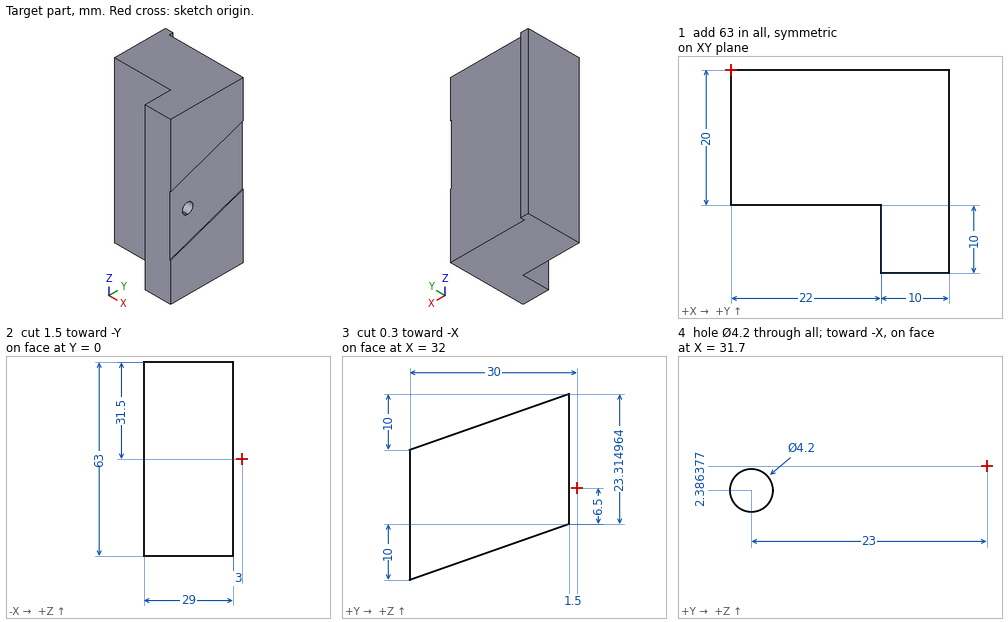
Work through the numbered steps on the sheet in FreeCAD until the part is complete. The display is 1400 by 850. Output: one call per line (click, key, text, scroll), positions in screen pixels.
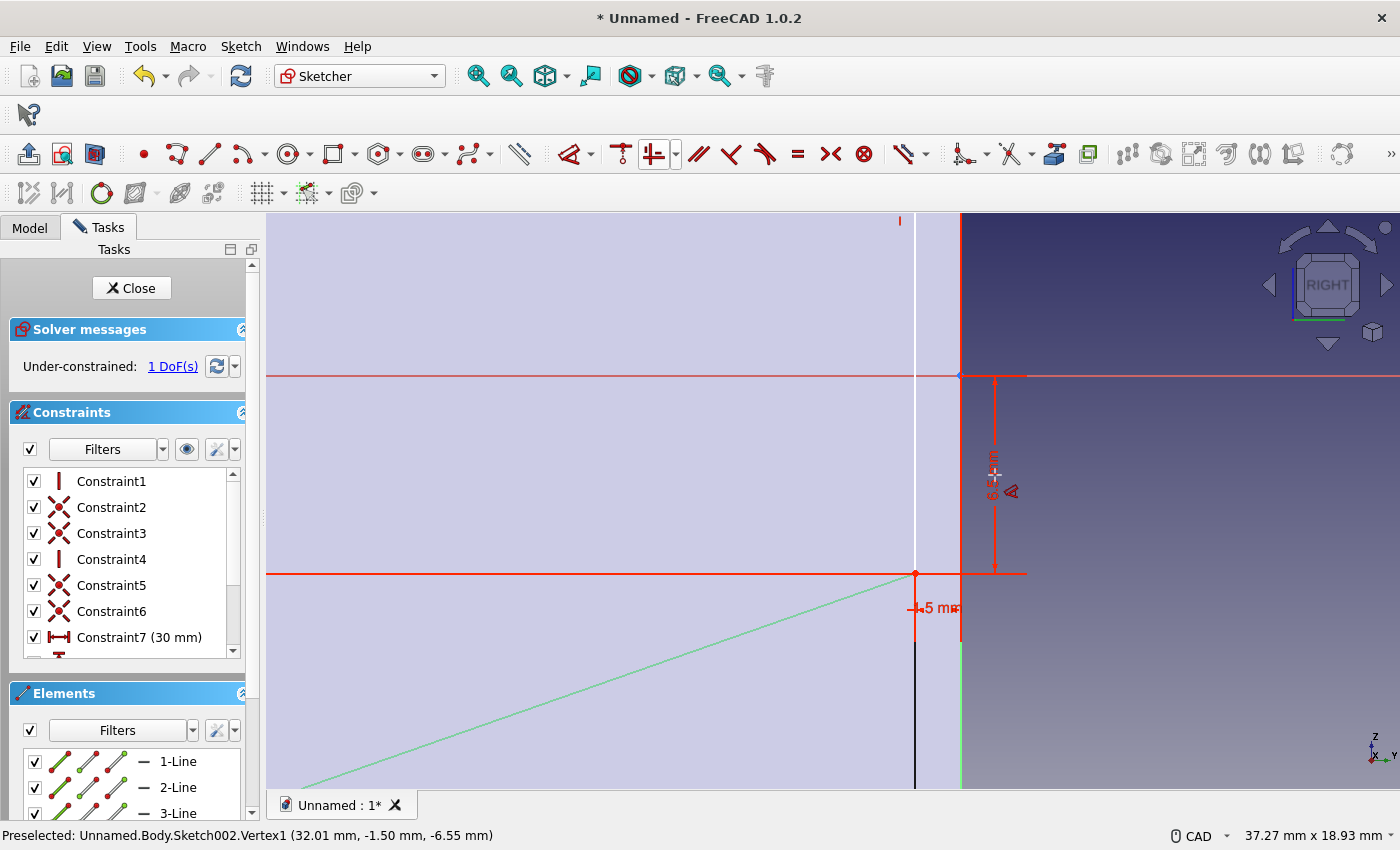
click(915, 362)
click(881, 407)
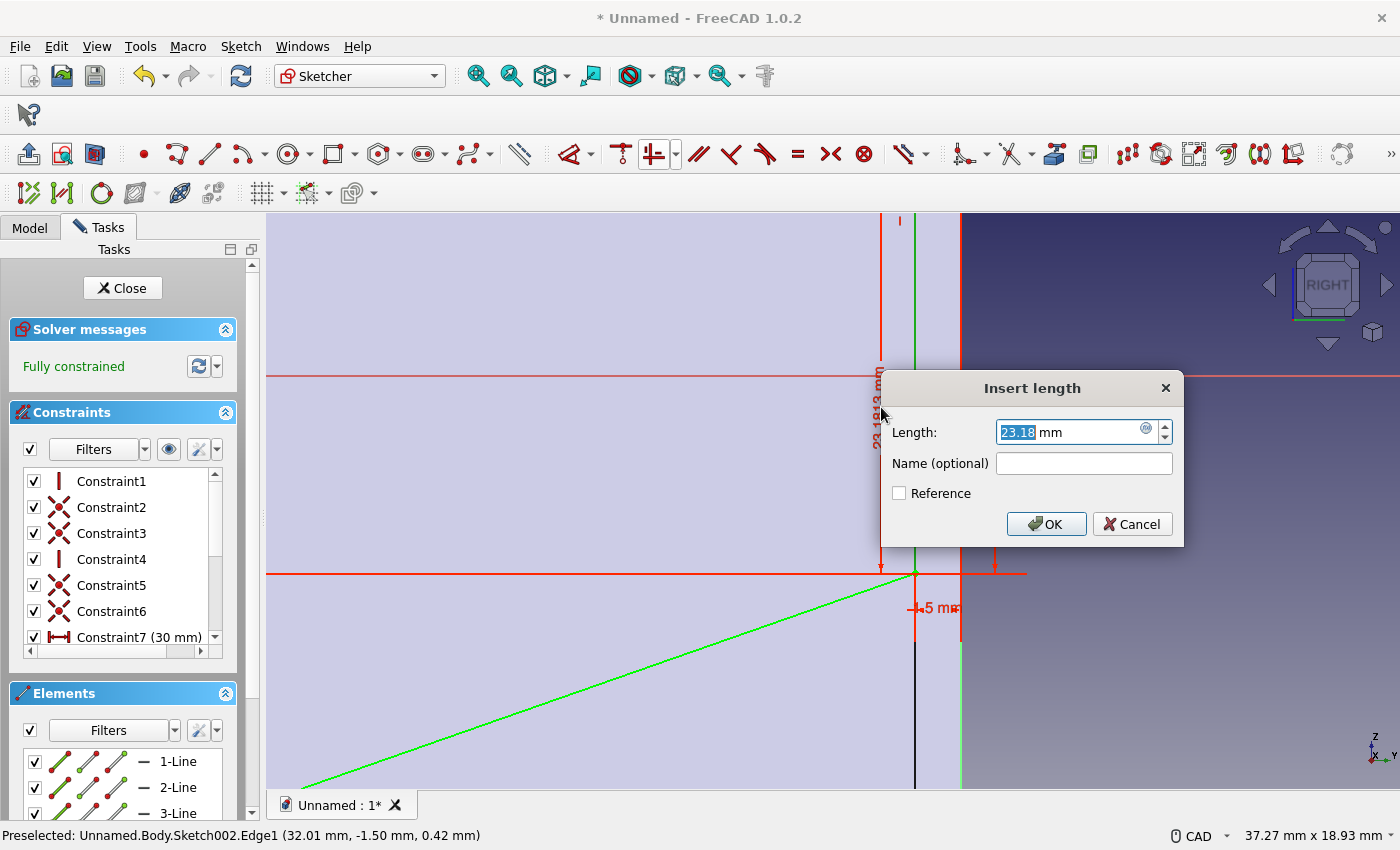
text(23.314964)
key(Return)
key(Escape)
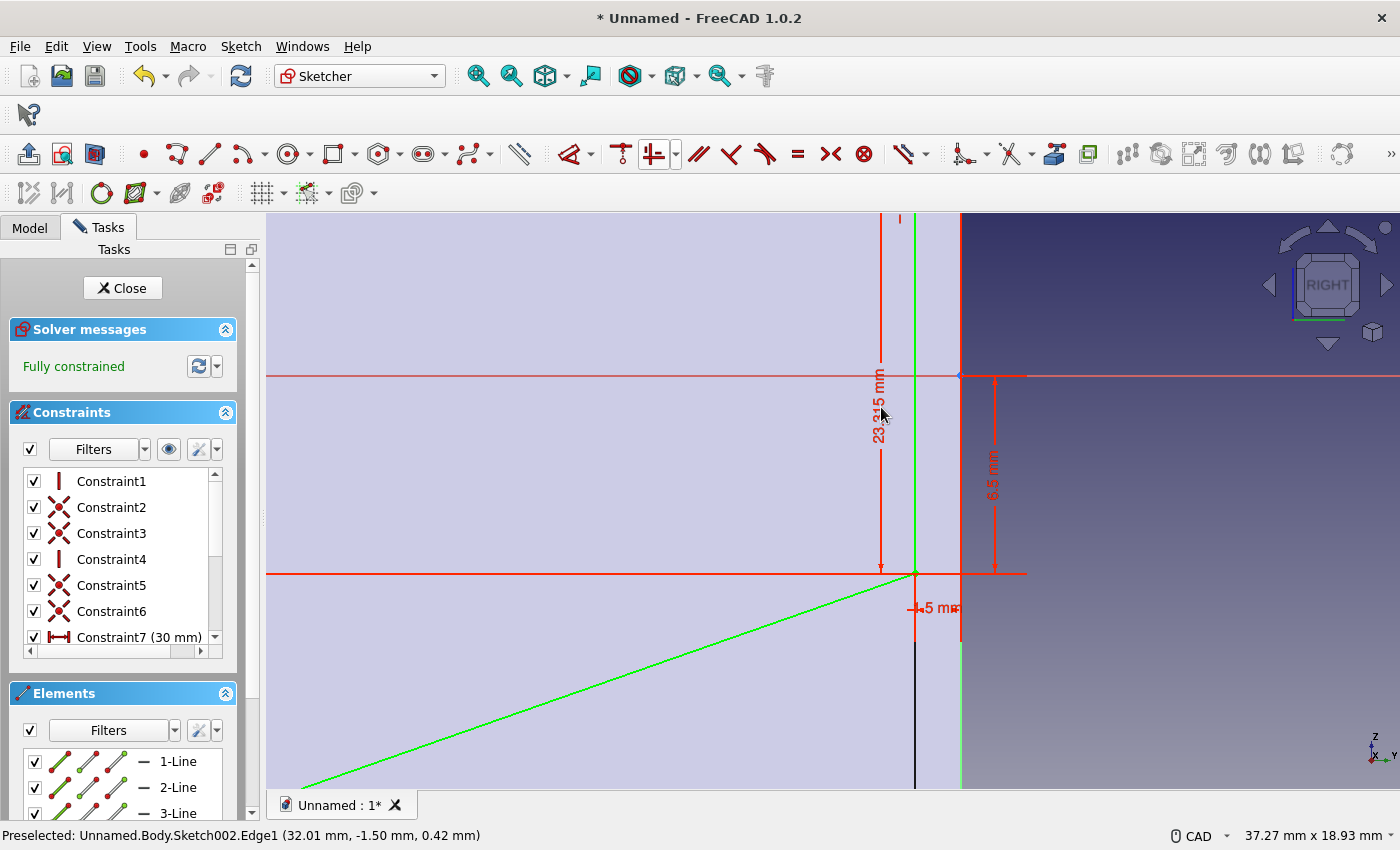
click(123, 288)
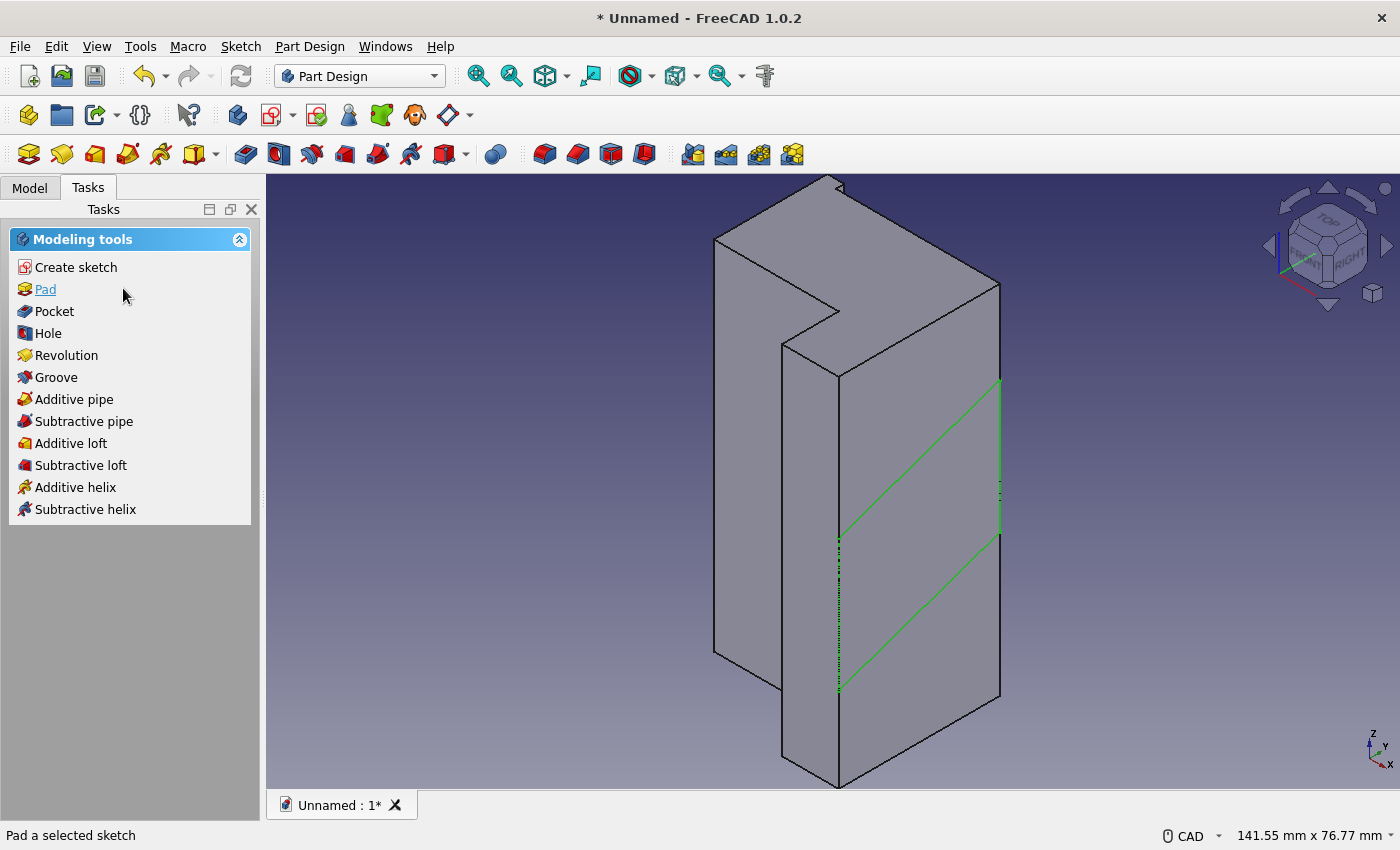
click(246, 154)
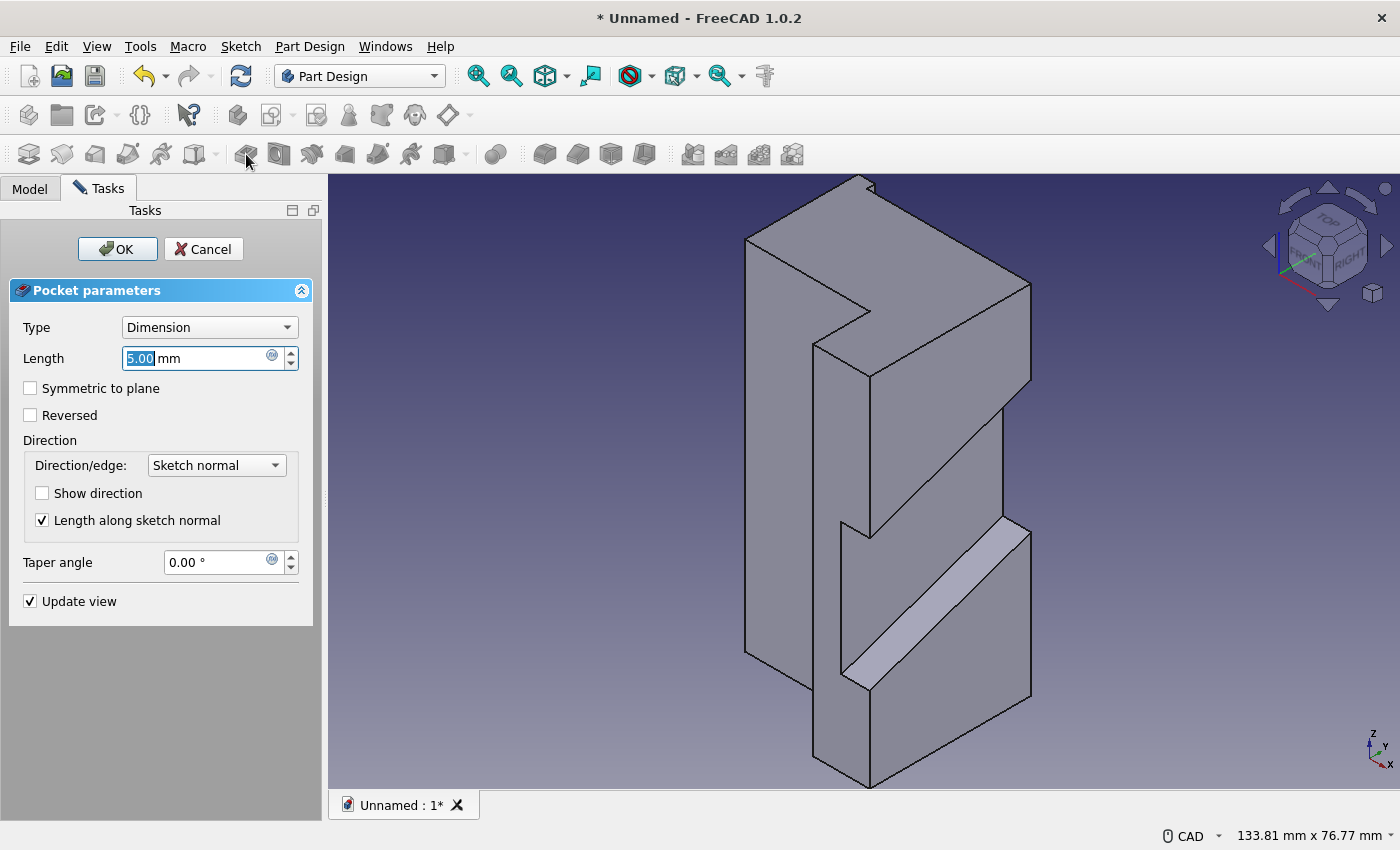
text(0.3)
key(Tab)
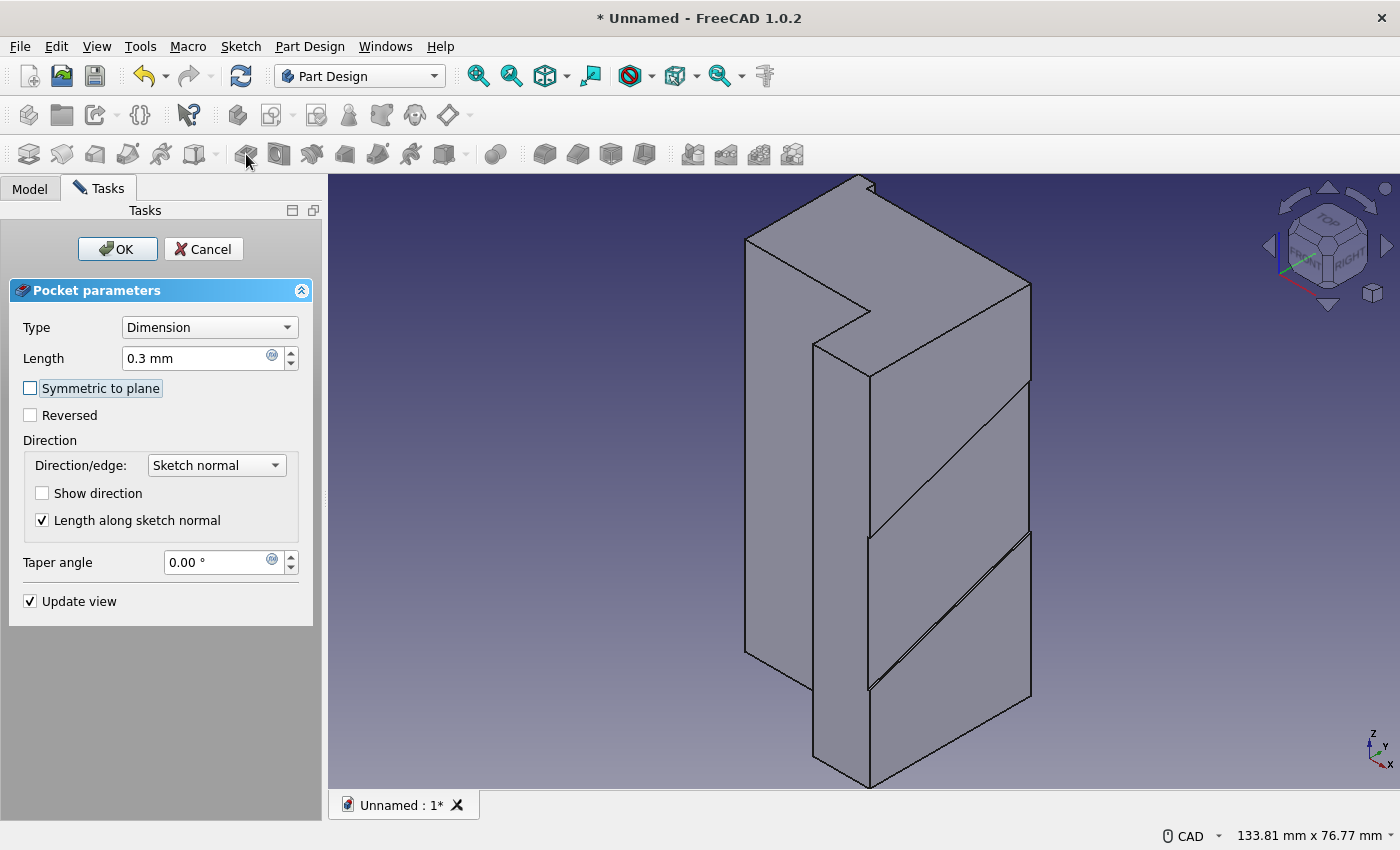
click(118, 249)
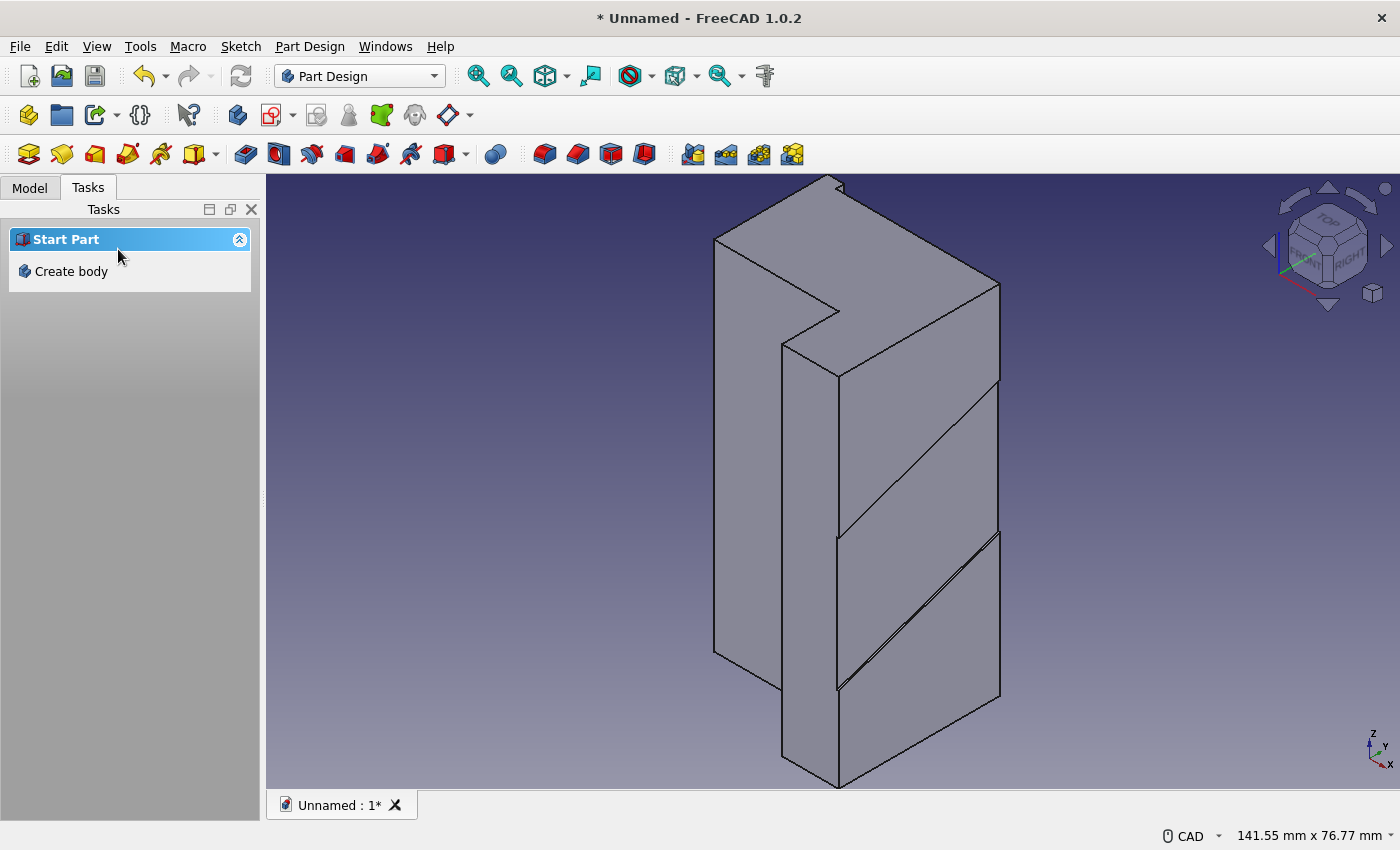
click(479, 76)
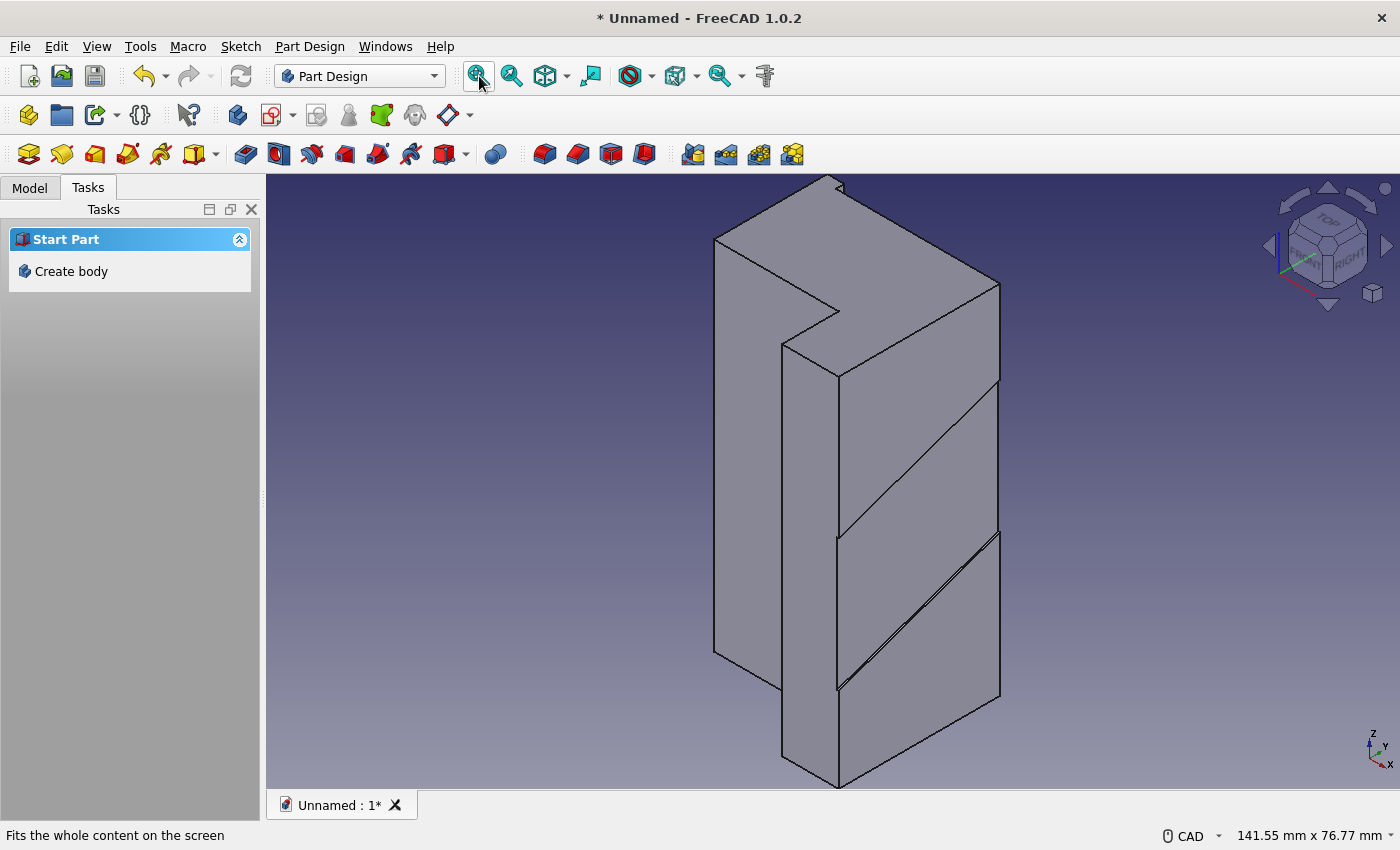
click(918, 533)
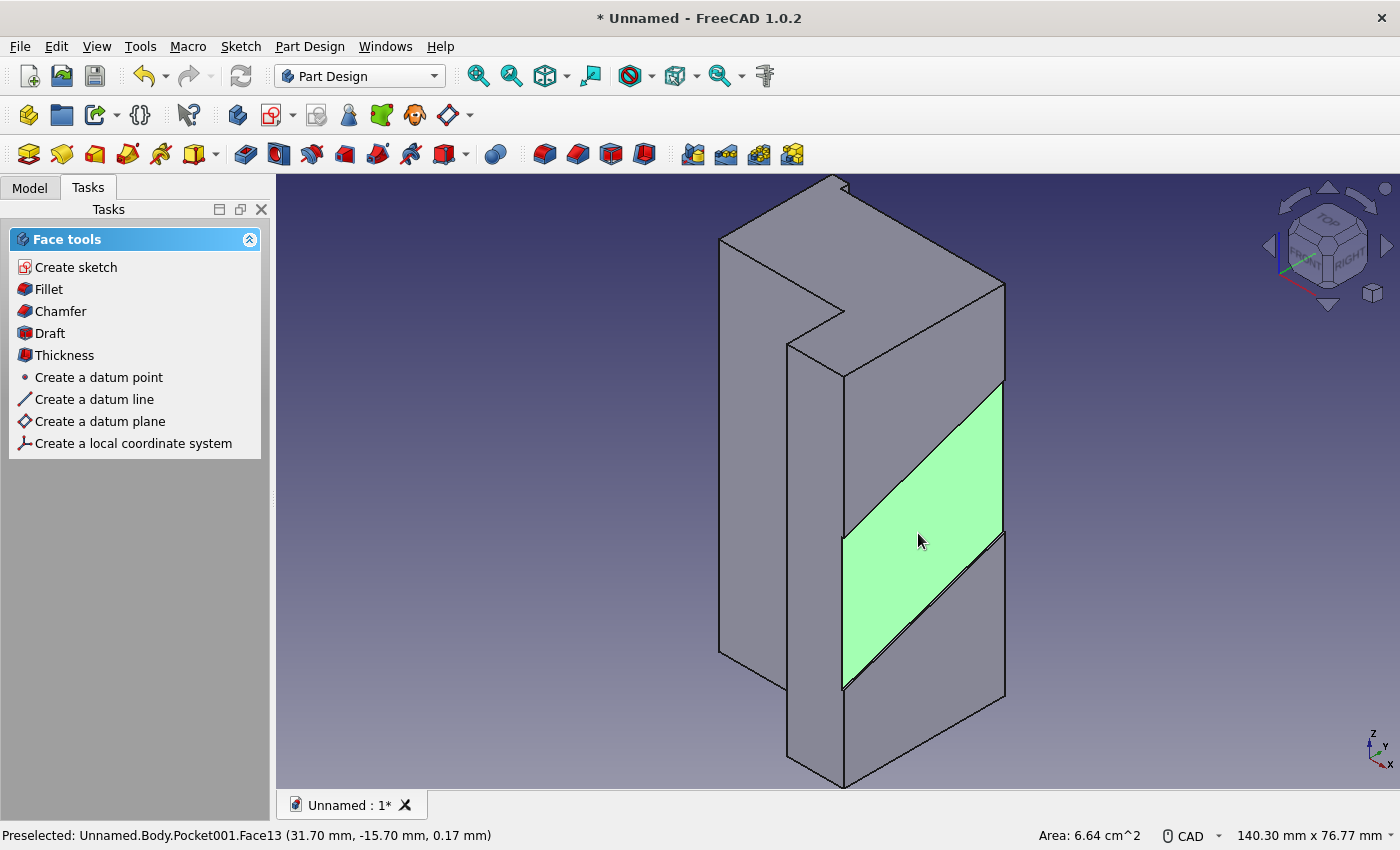
click(270, 116)